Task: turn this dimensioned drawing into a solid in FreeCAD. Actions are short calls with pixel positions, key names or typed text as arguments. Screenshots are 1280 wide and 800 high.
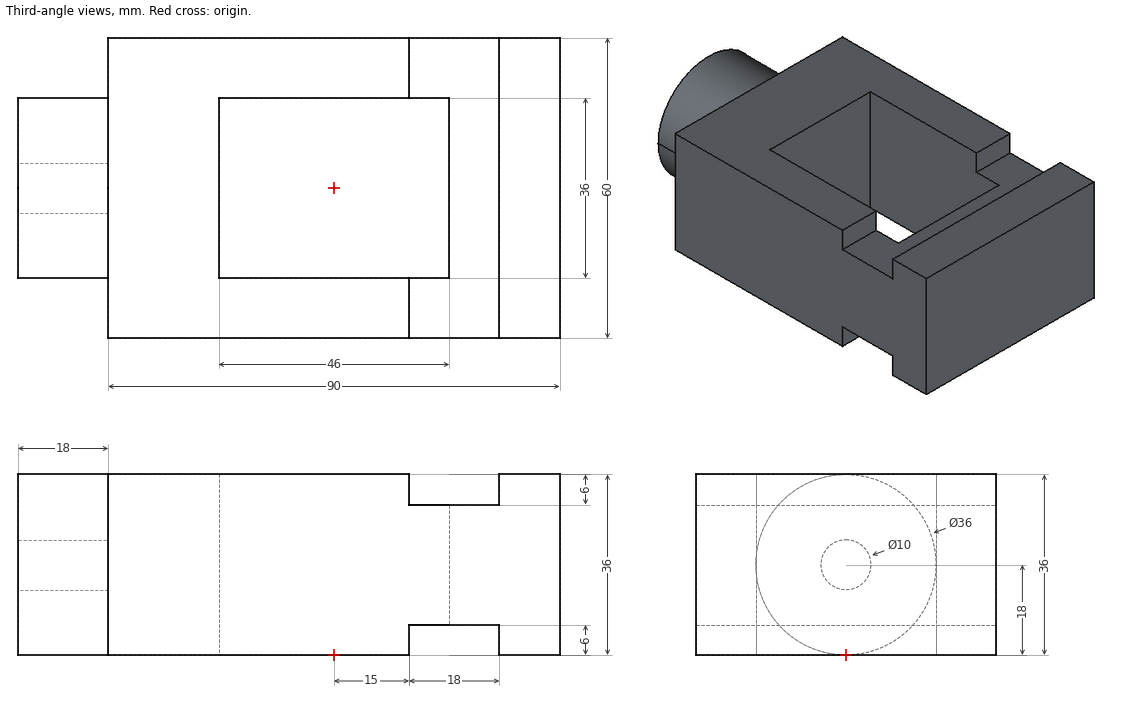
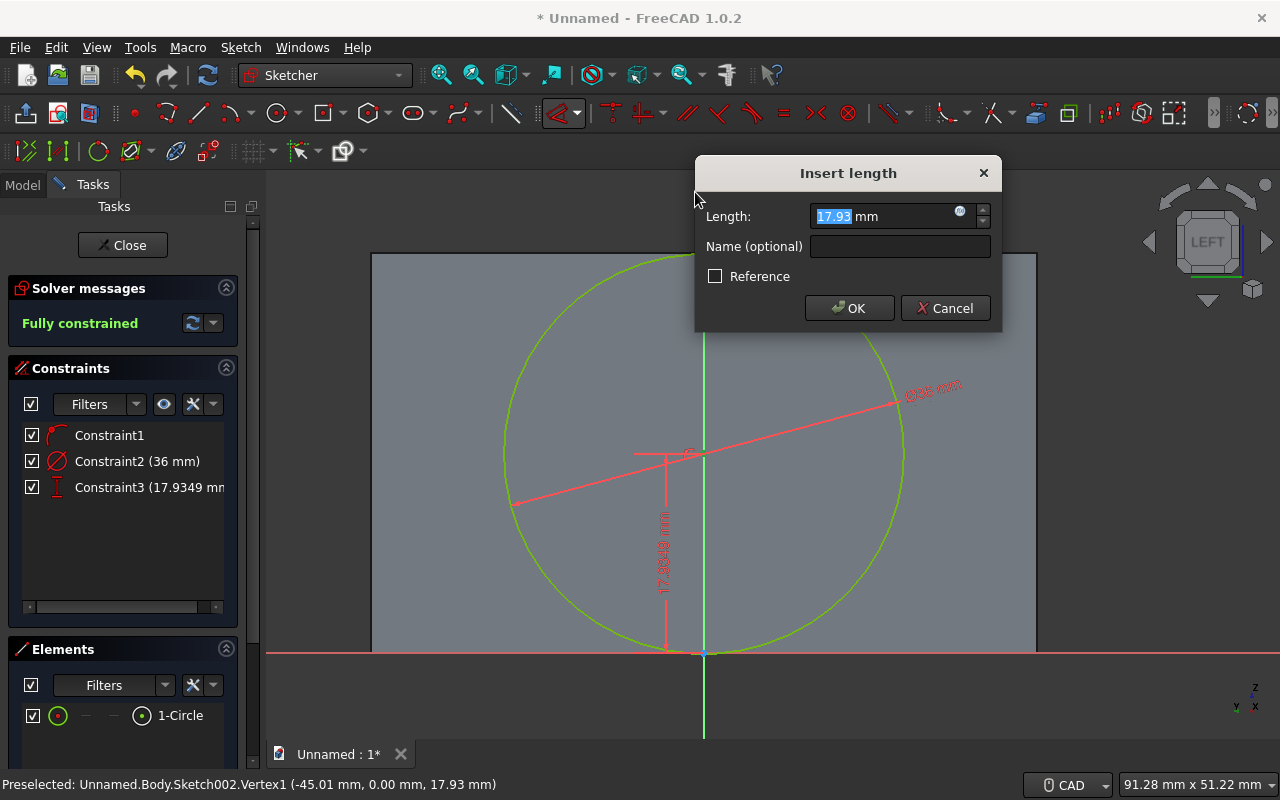
text(18)
key(Return)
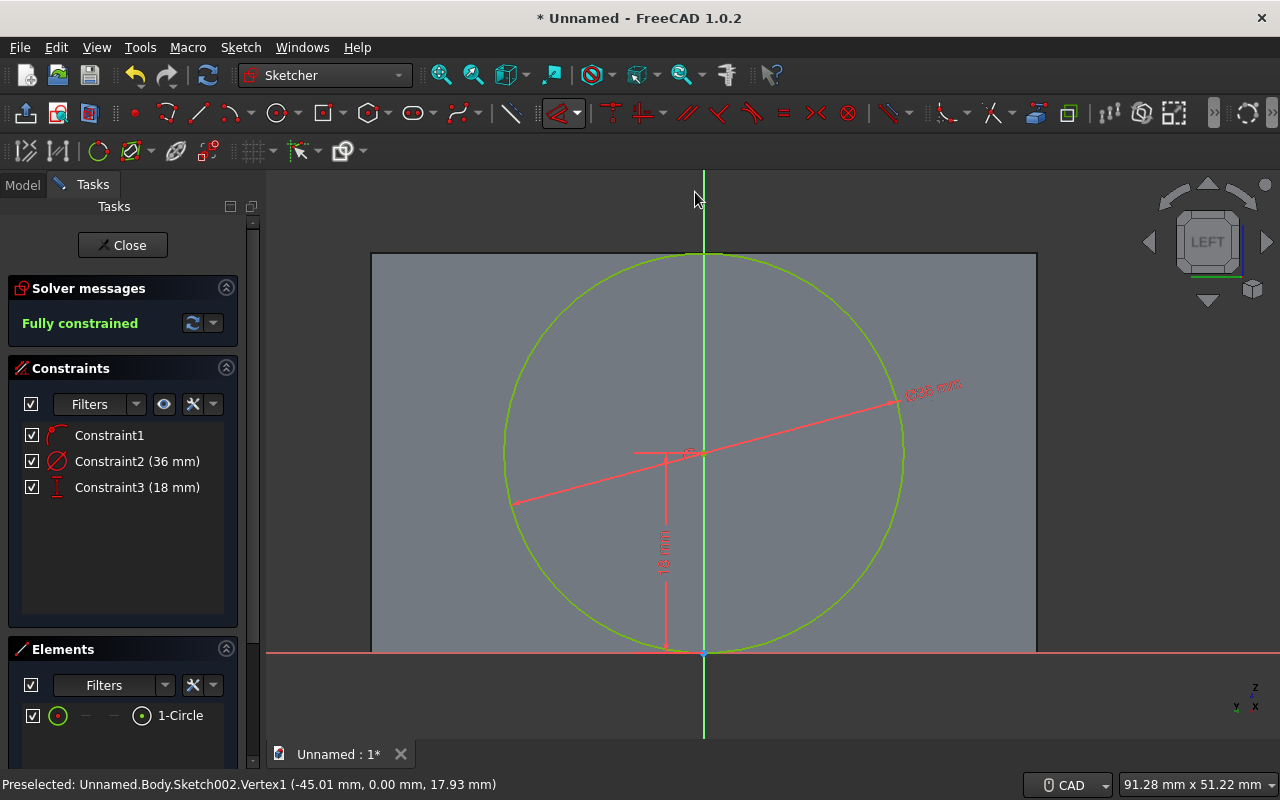
click(123, 245)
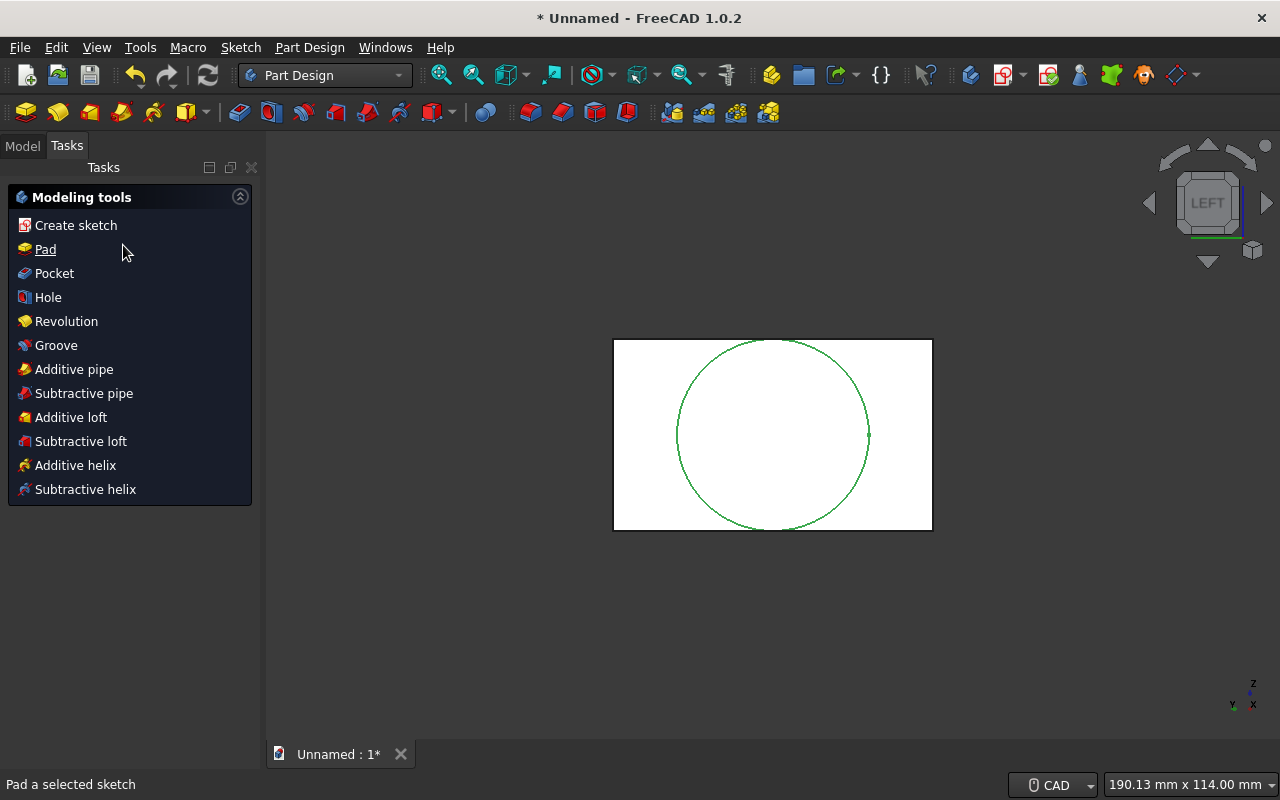
click(26, 112)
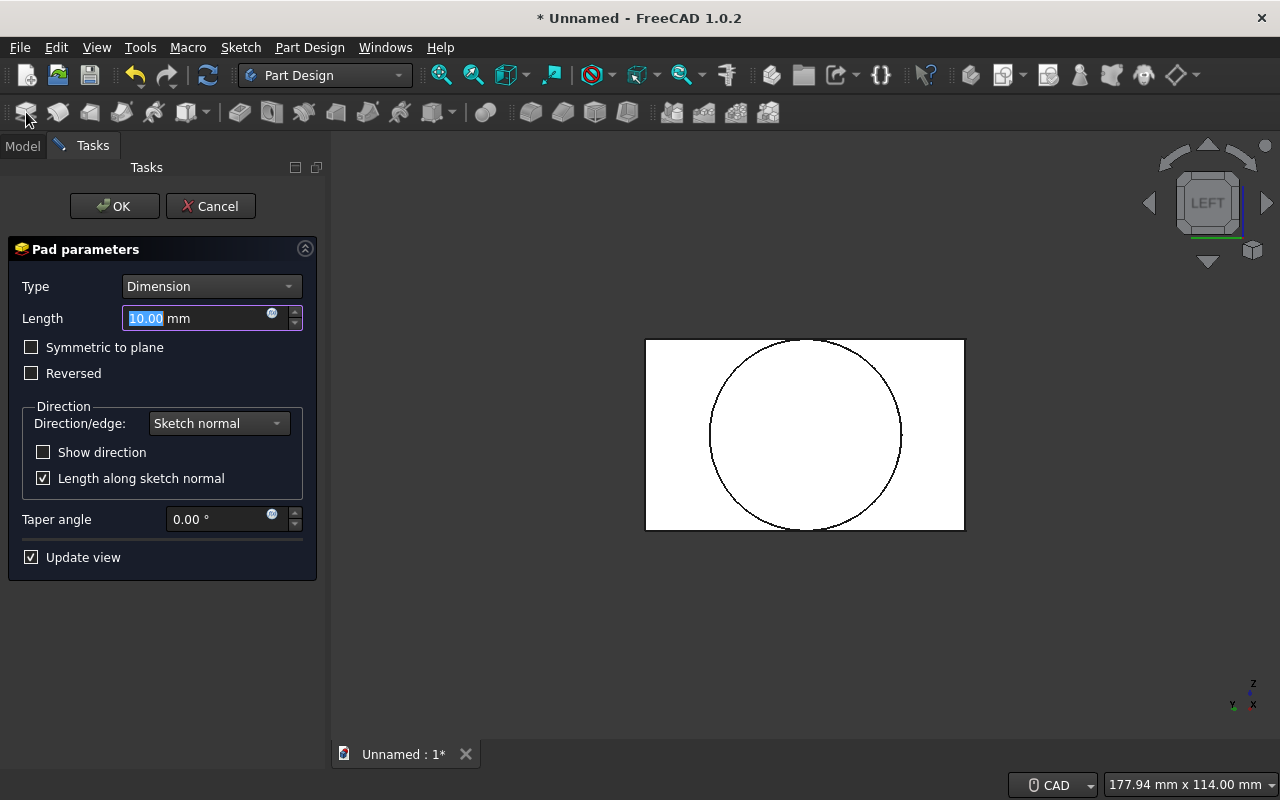
text(18)
key(Tab)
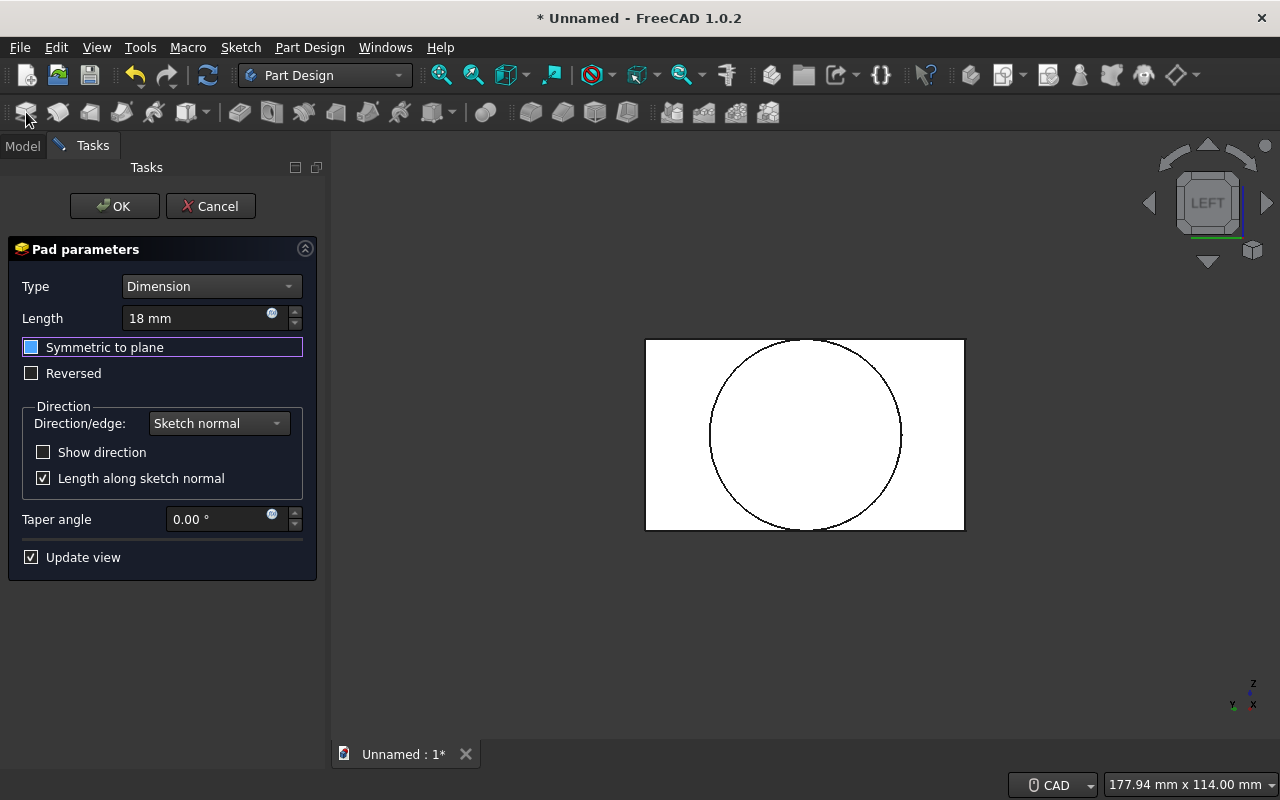
click(115, 206)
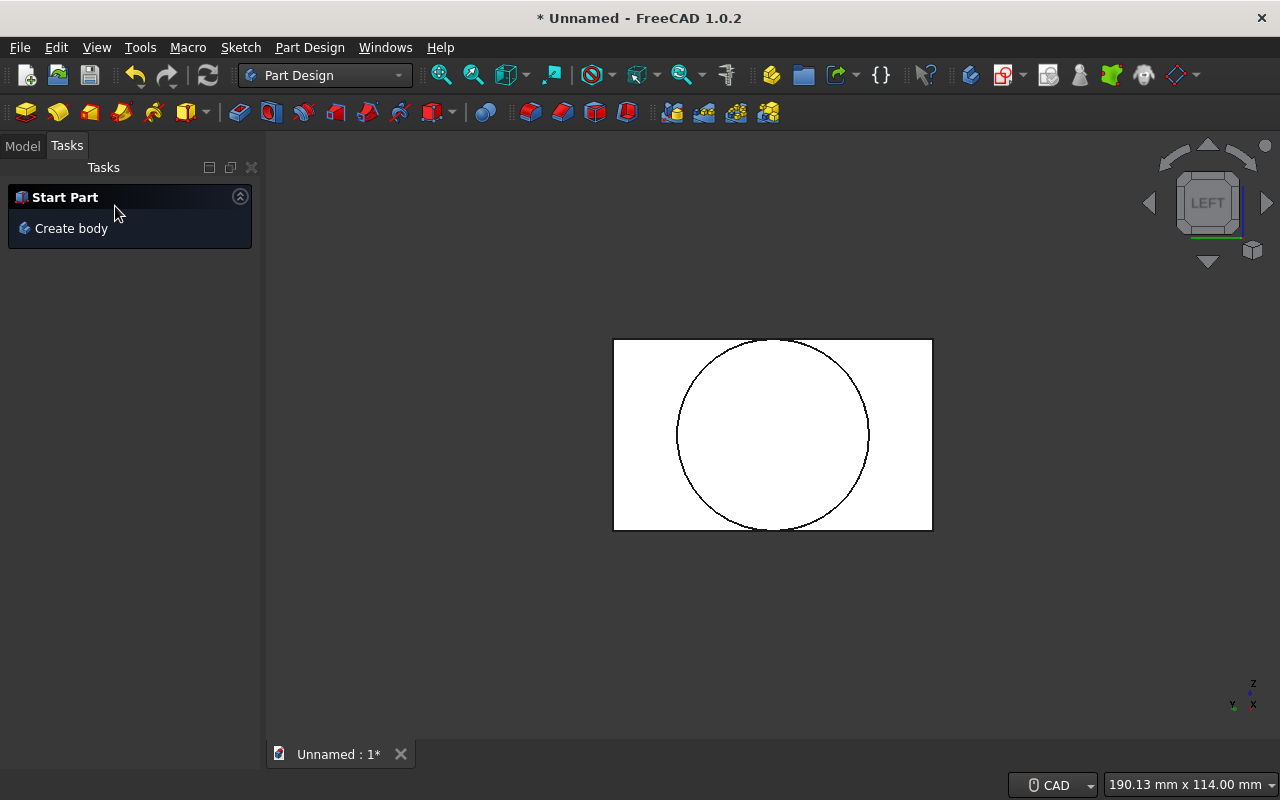
click(442, 76)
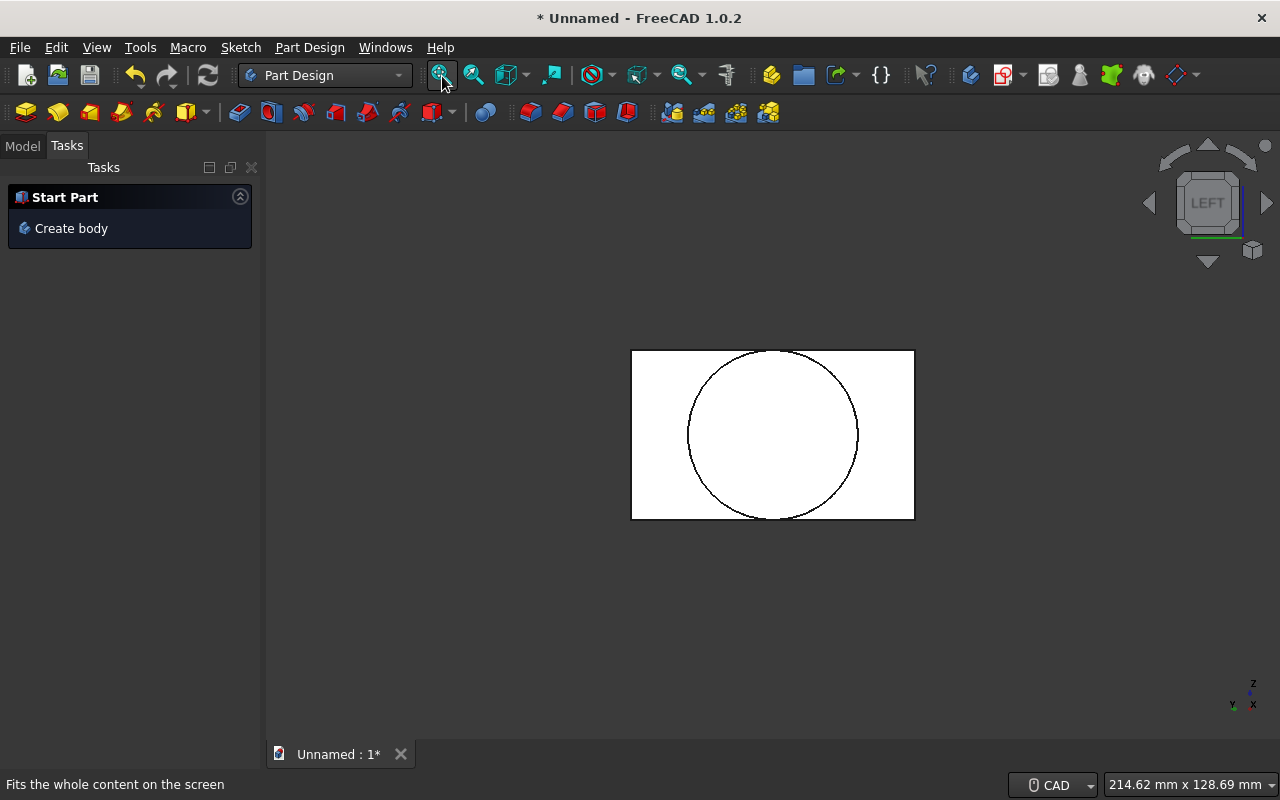
click(773, 434)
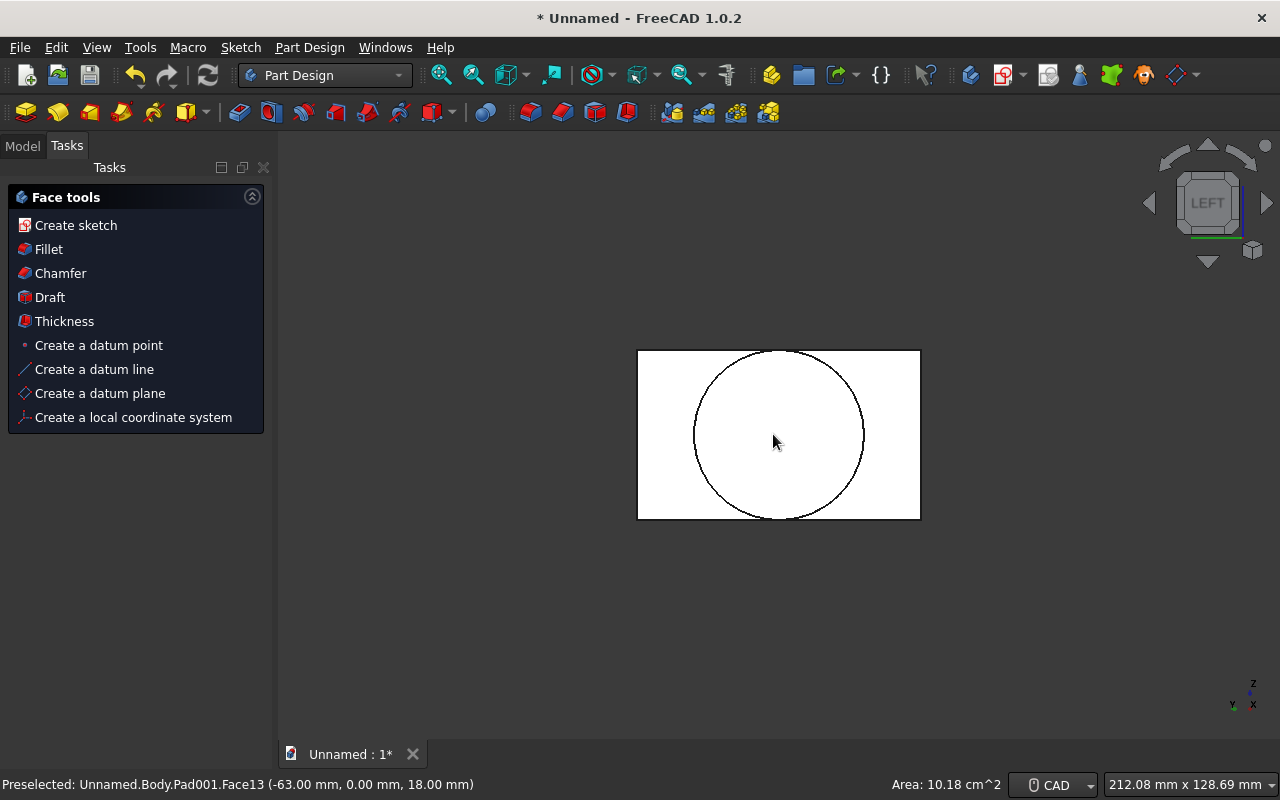
click(1004, 76)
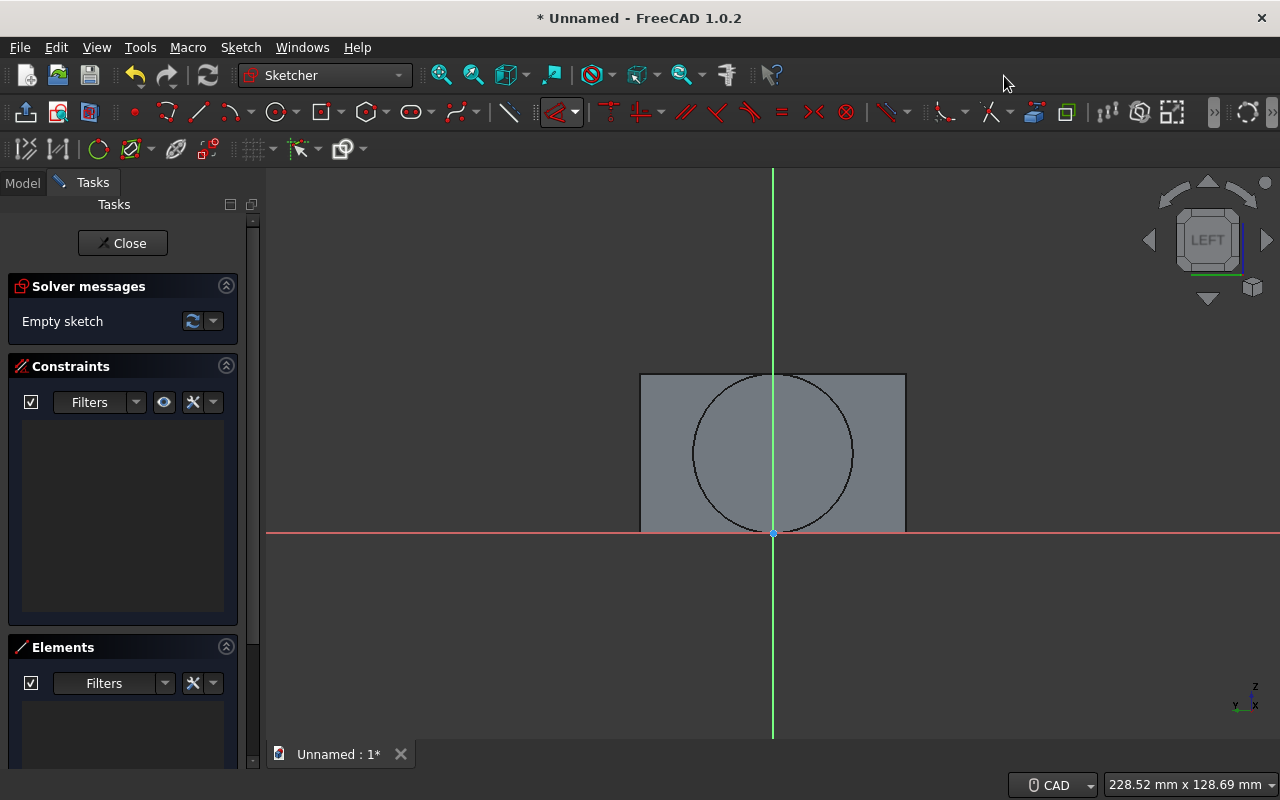
scroll(803, 495, up, 6)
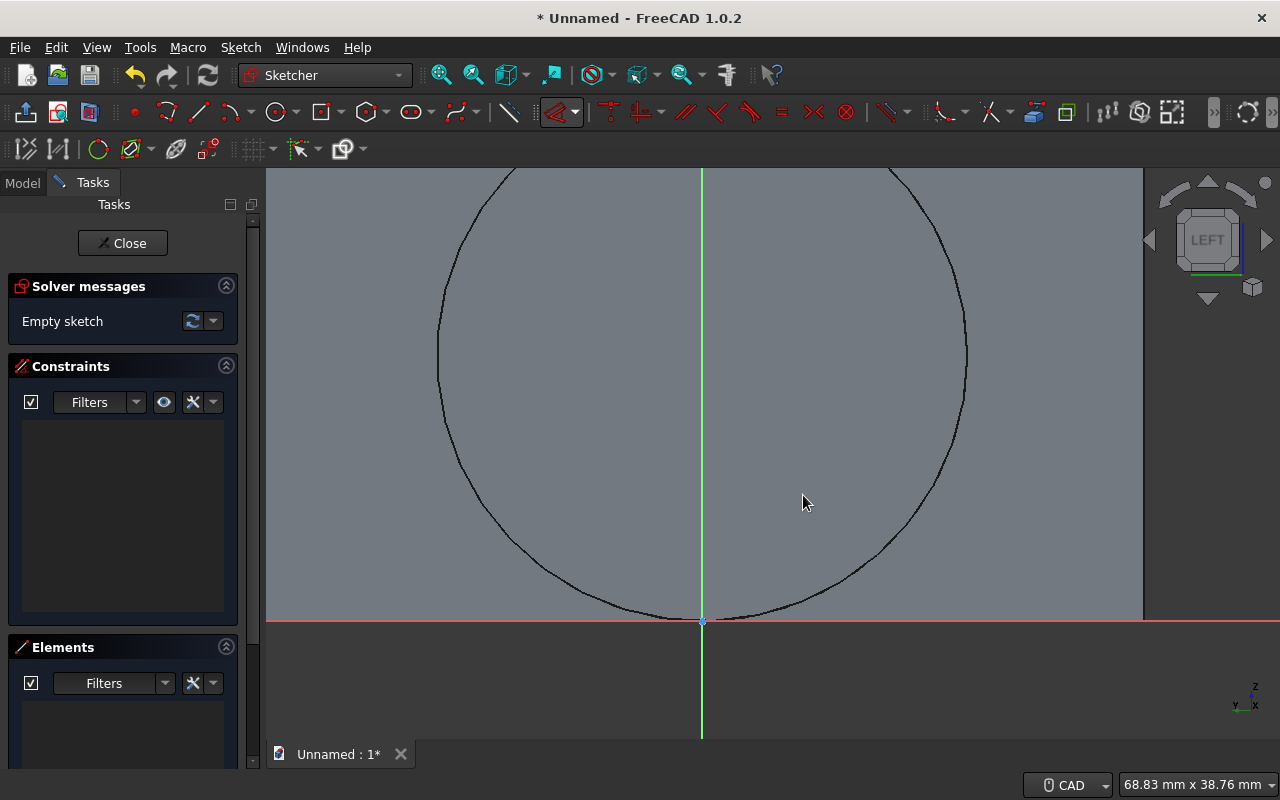
click(276, 112)